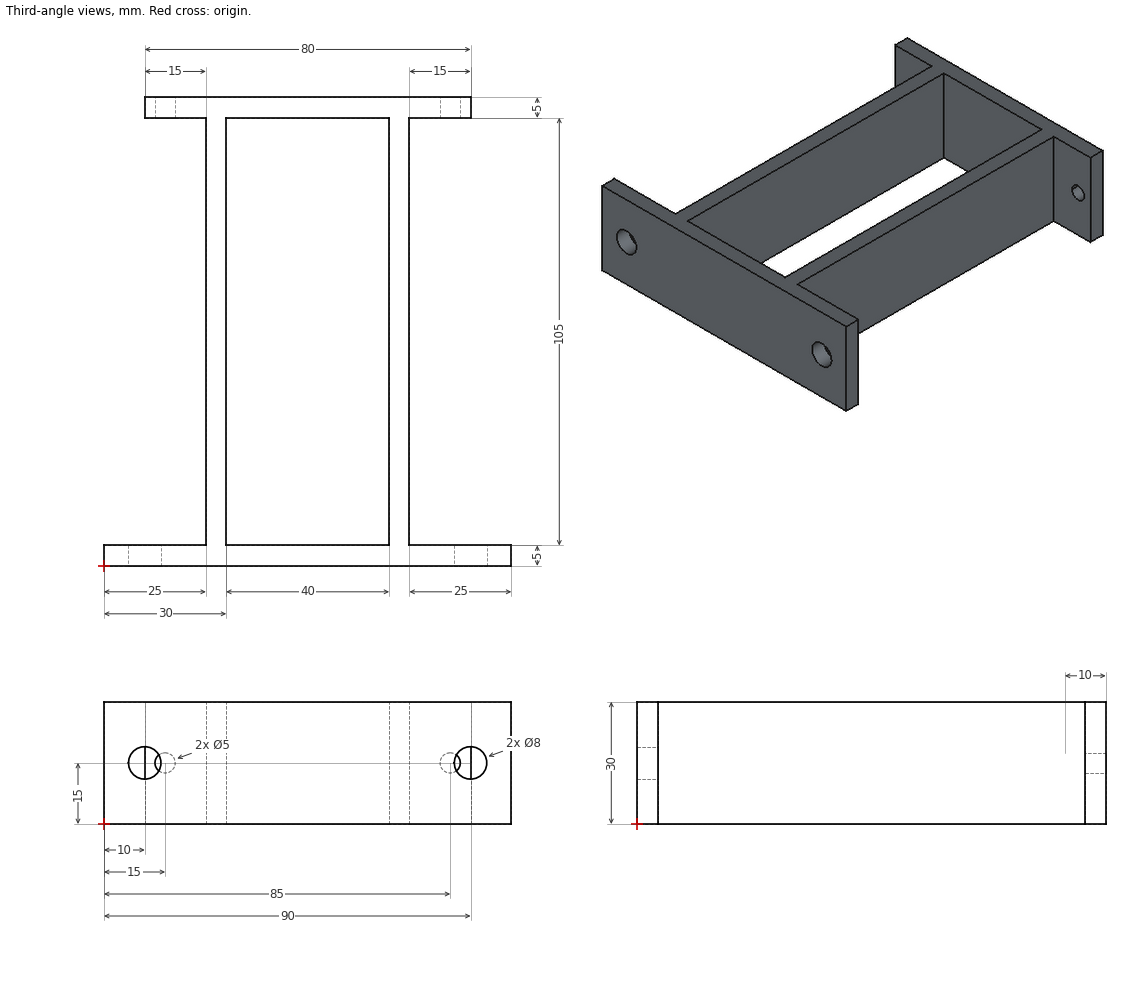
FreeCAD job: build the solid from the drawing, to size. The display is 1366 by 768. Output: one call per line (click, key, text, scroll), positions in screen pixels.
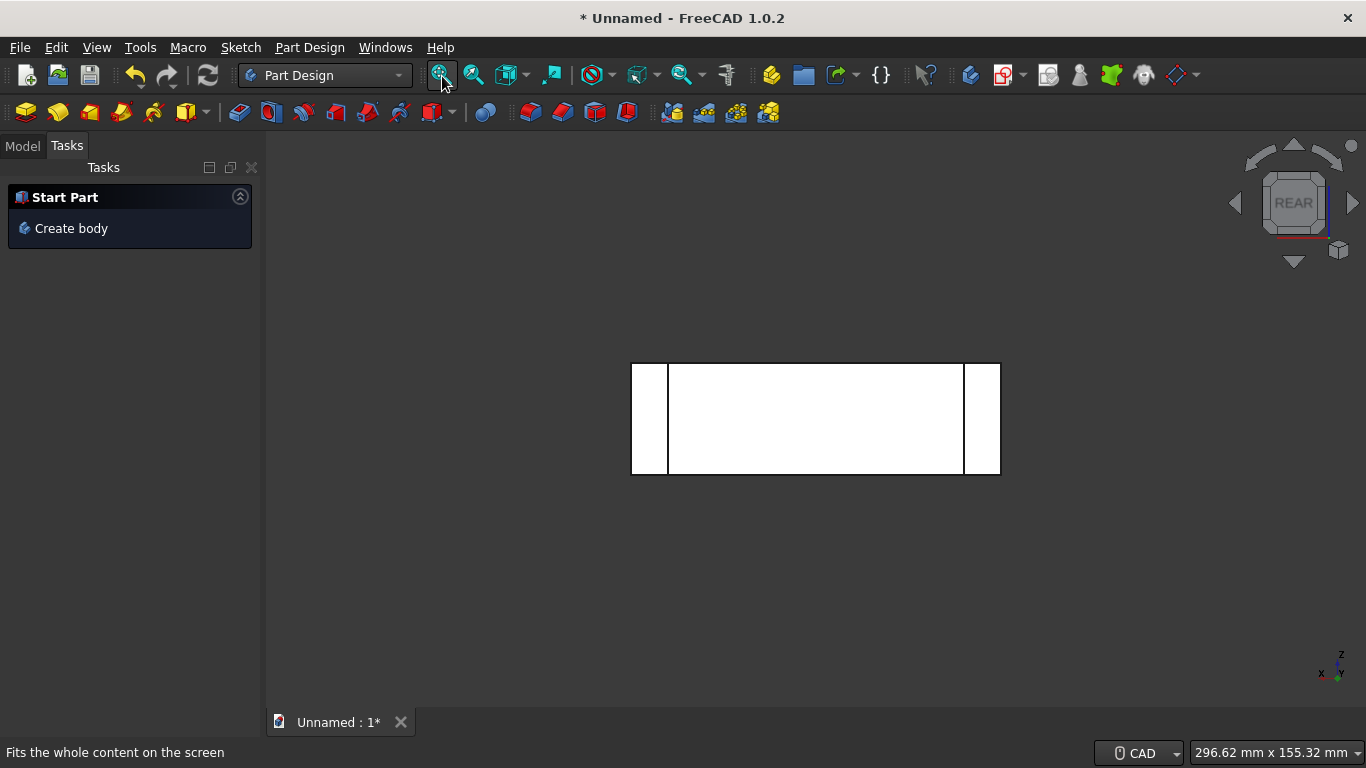
click(442, 76)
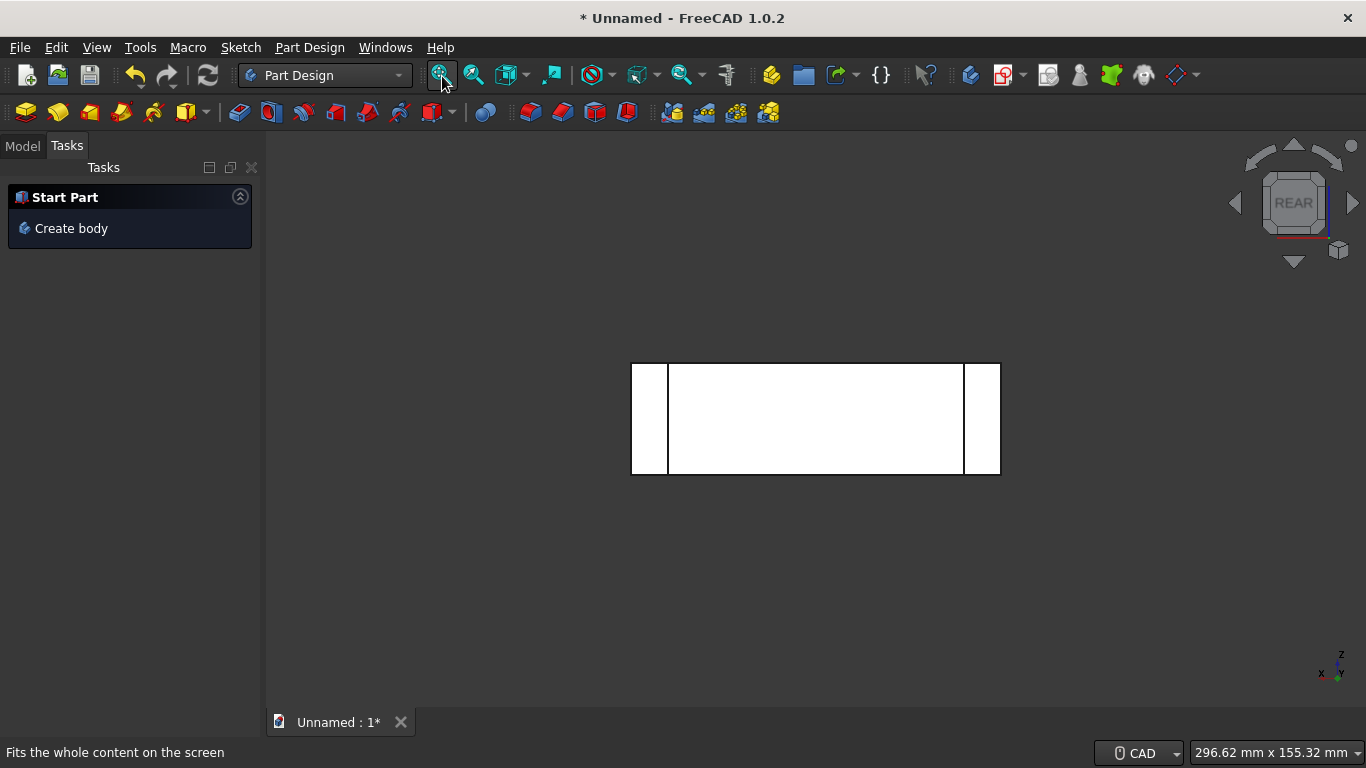
key(2)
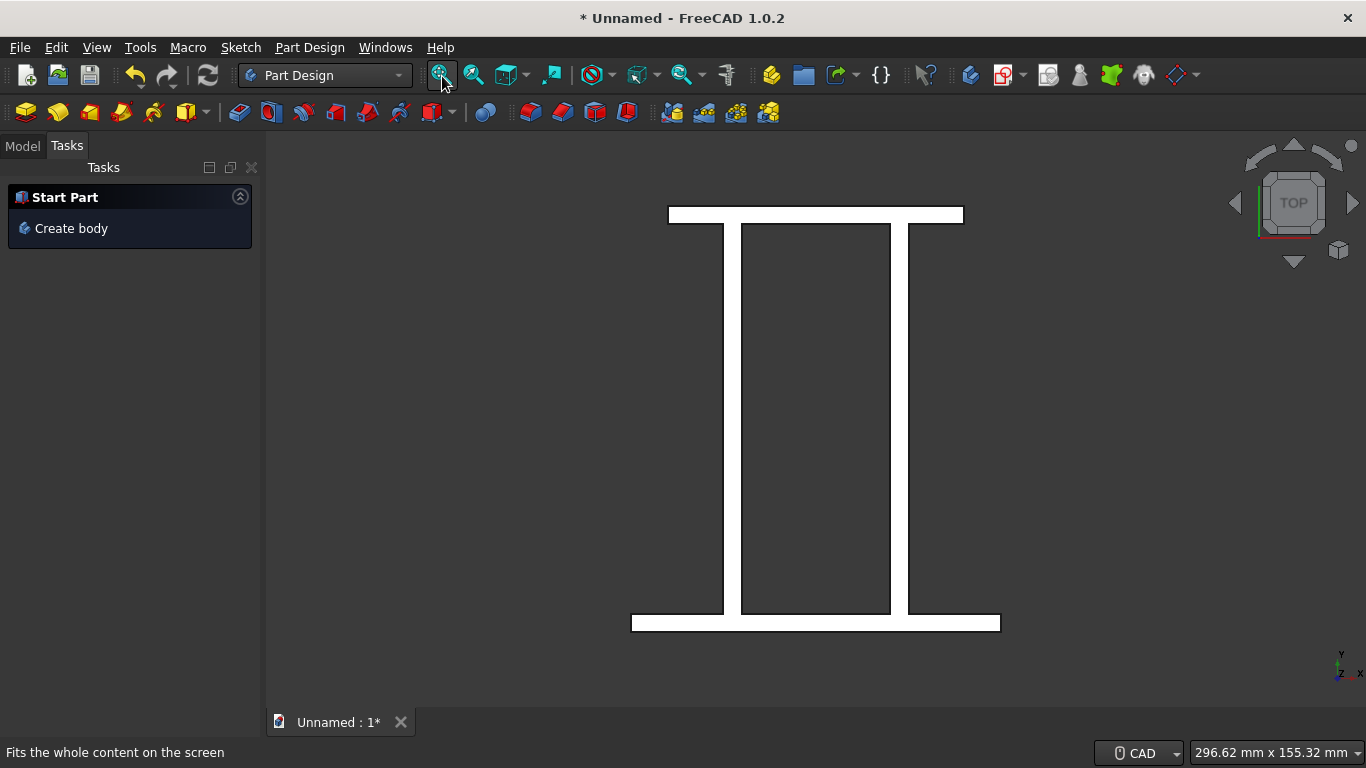
key(3)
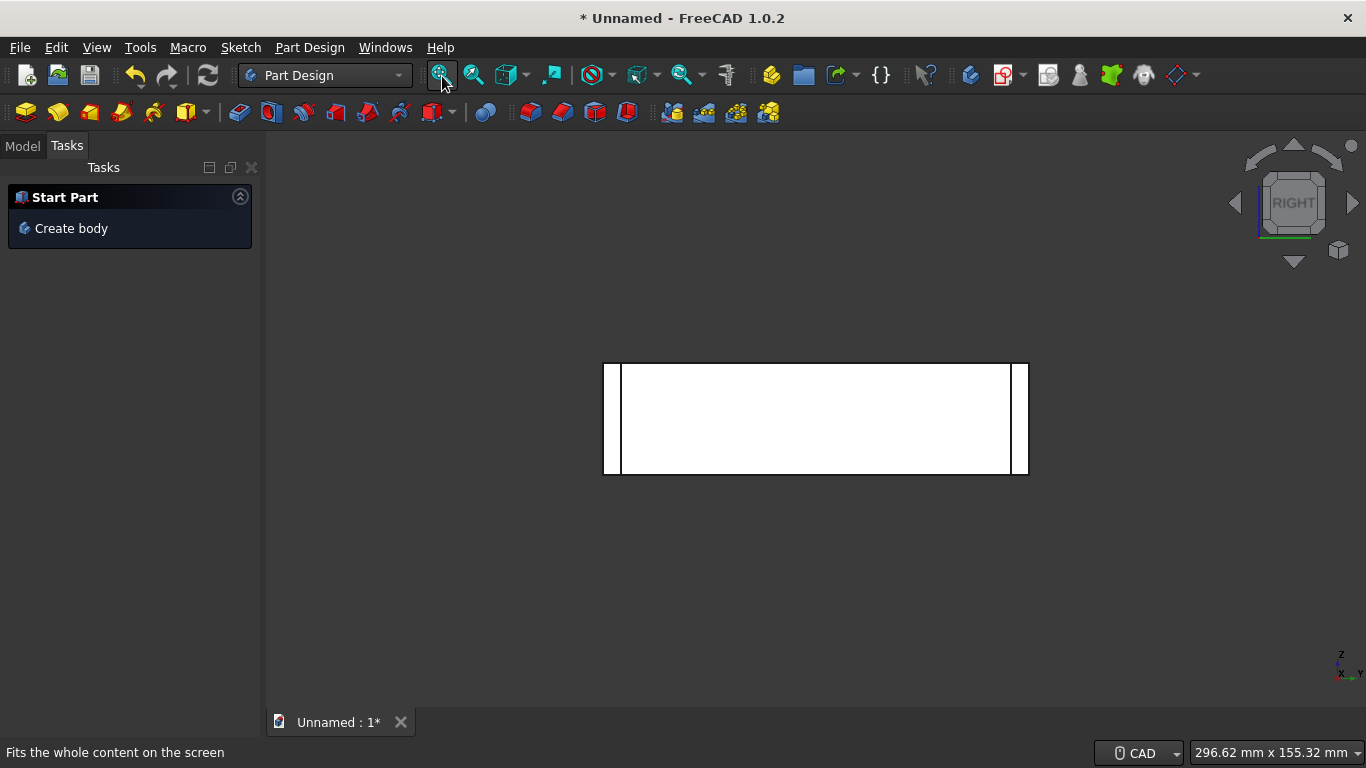
click(442, 76)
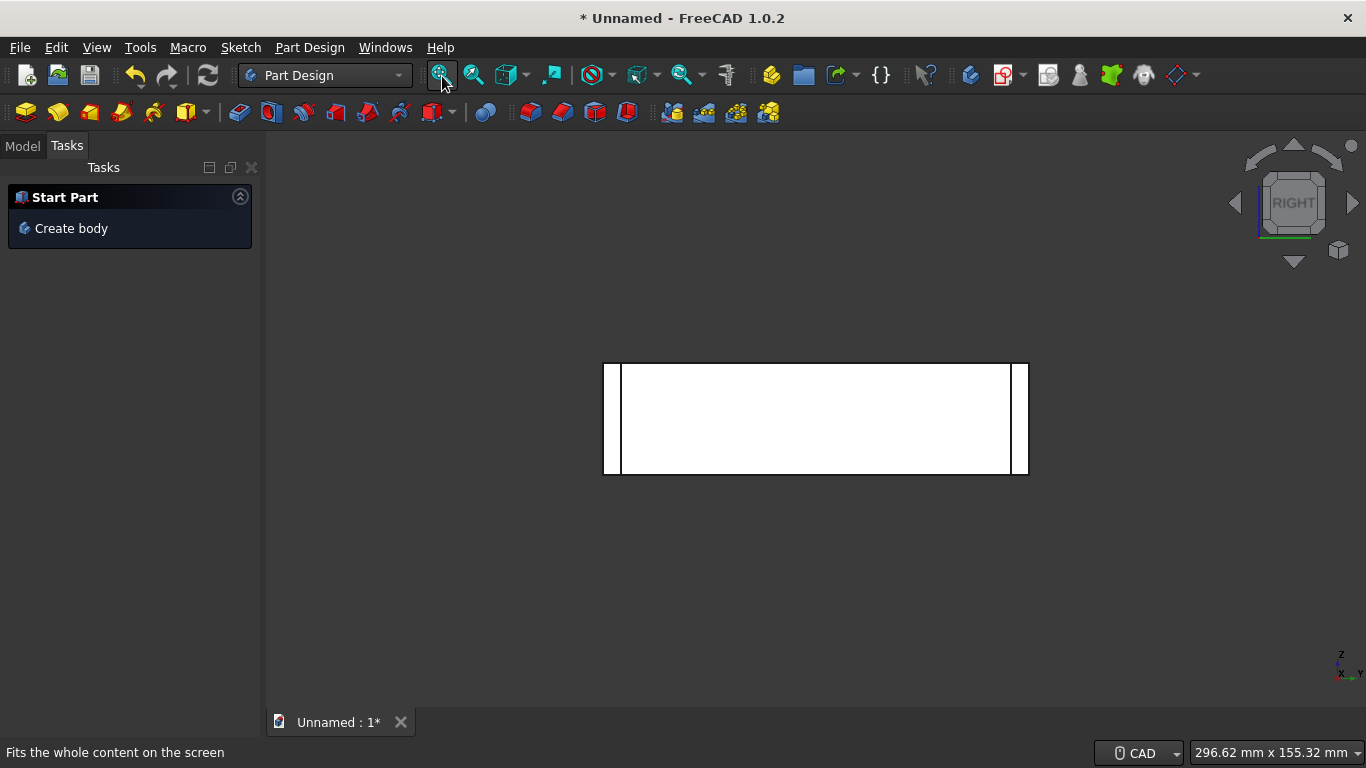
click(23, 145)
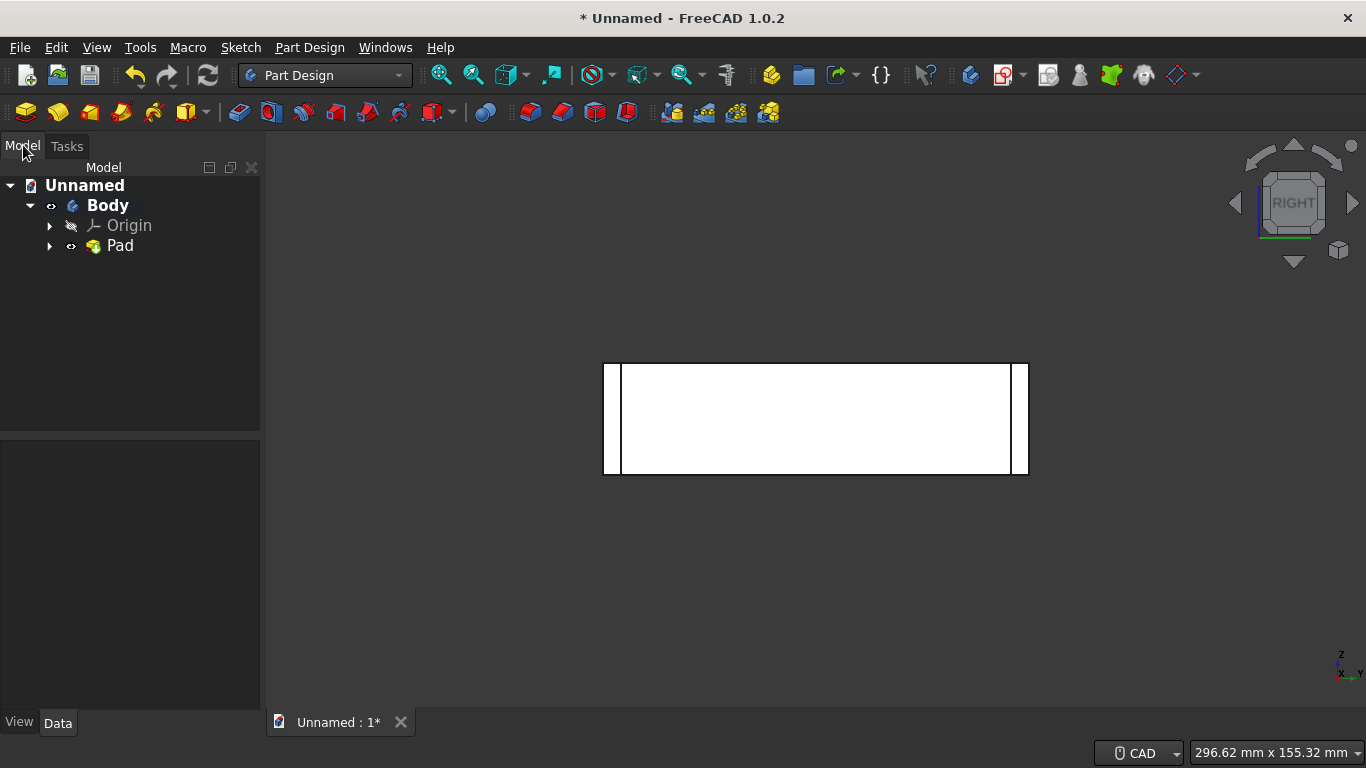
click(50, 226)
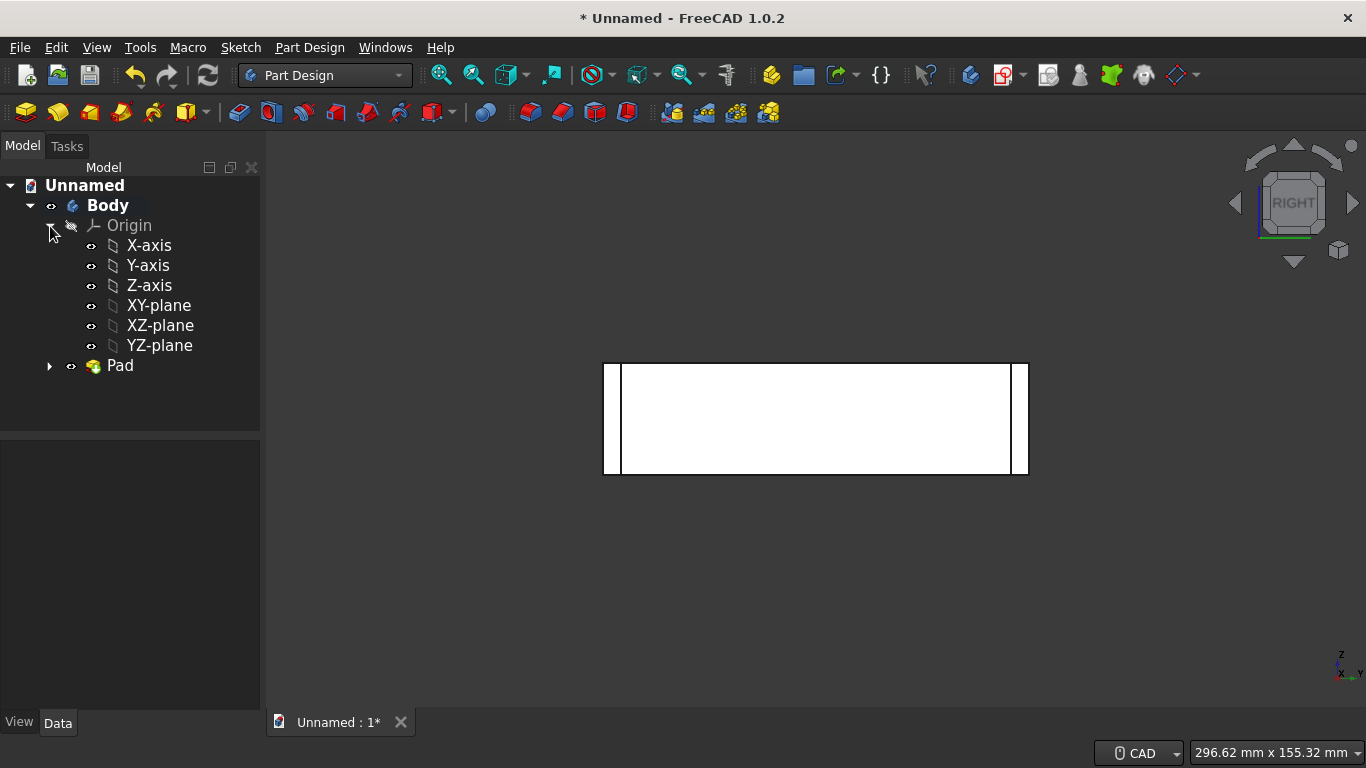
click(136, 326)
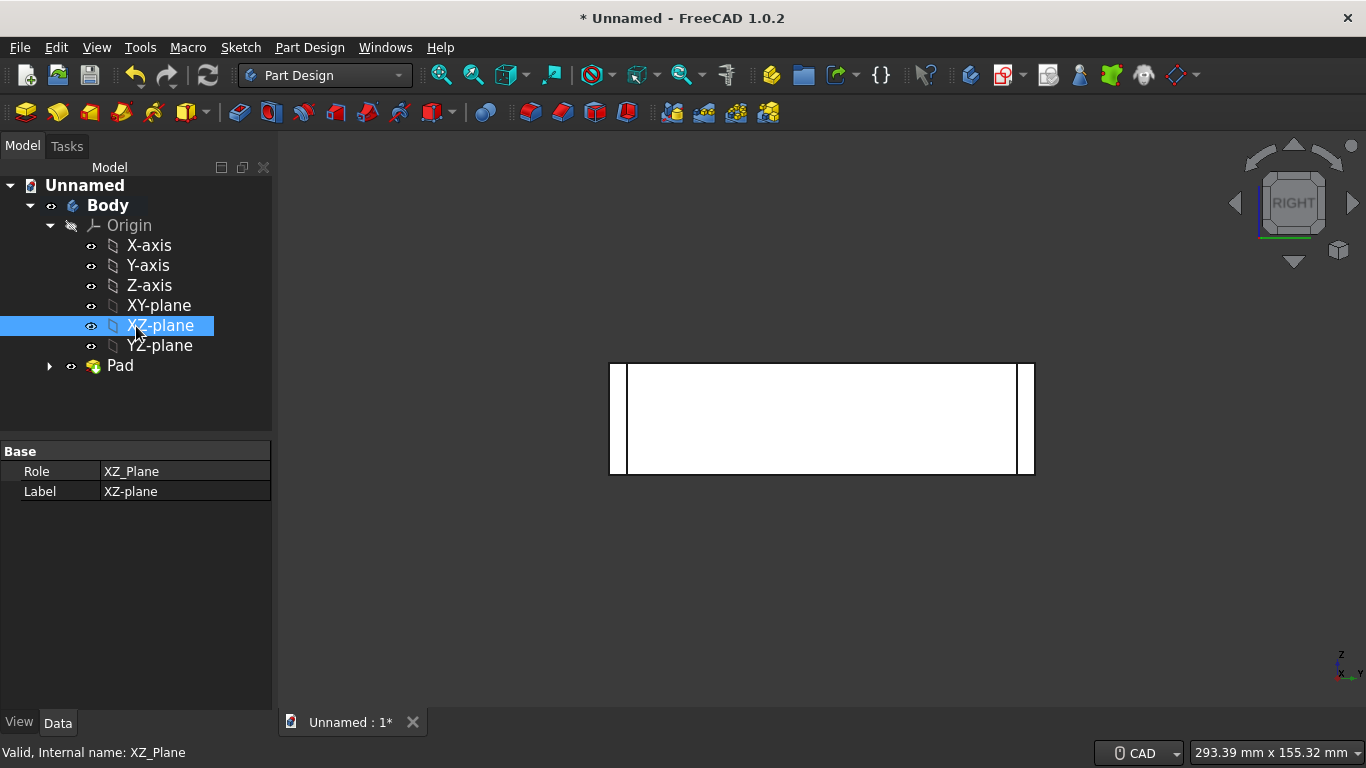
click(1176, 76)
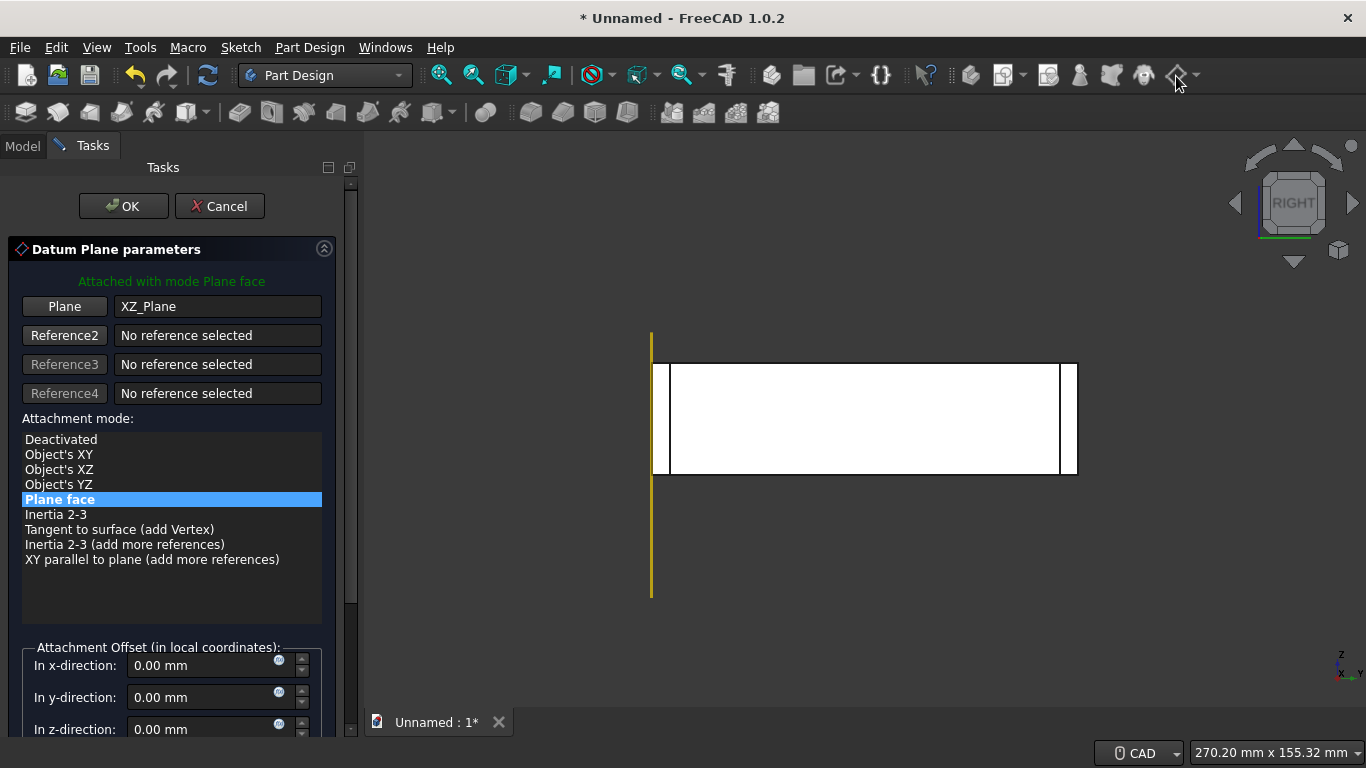
scroll(351, 456, down, 2)